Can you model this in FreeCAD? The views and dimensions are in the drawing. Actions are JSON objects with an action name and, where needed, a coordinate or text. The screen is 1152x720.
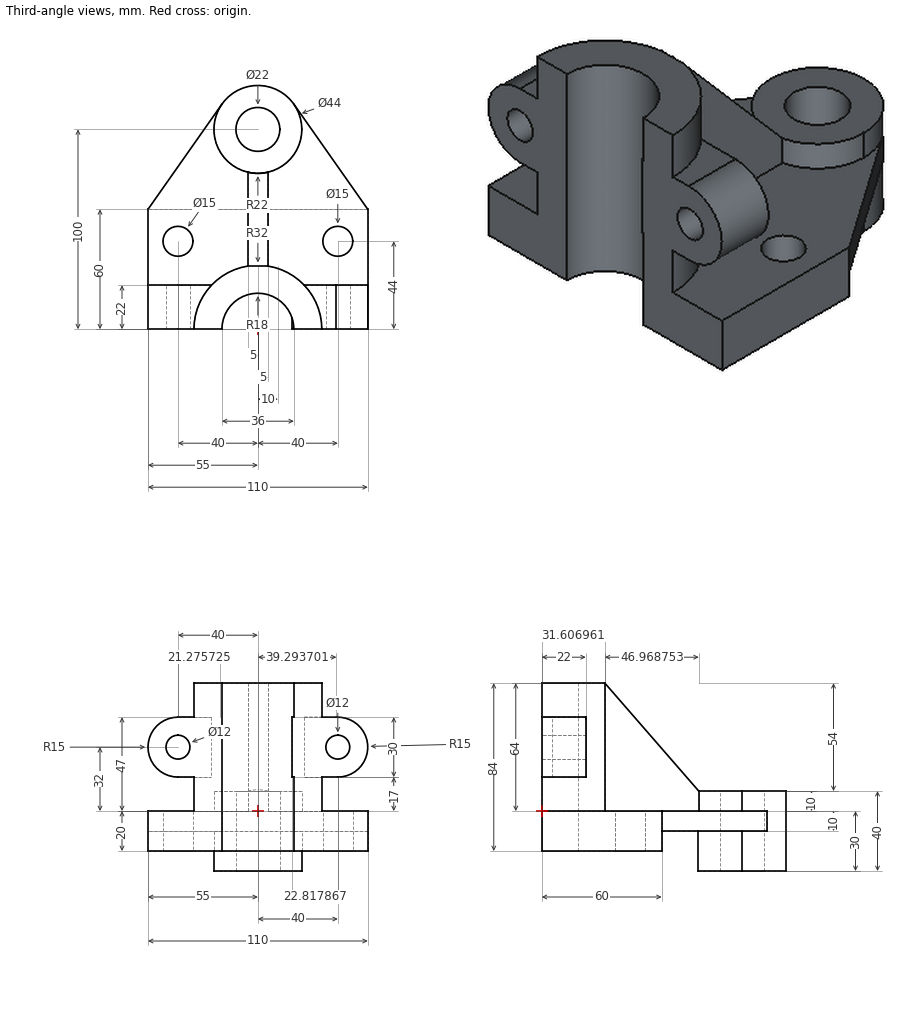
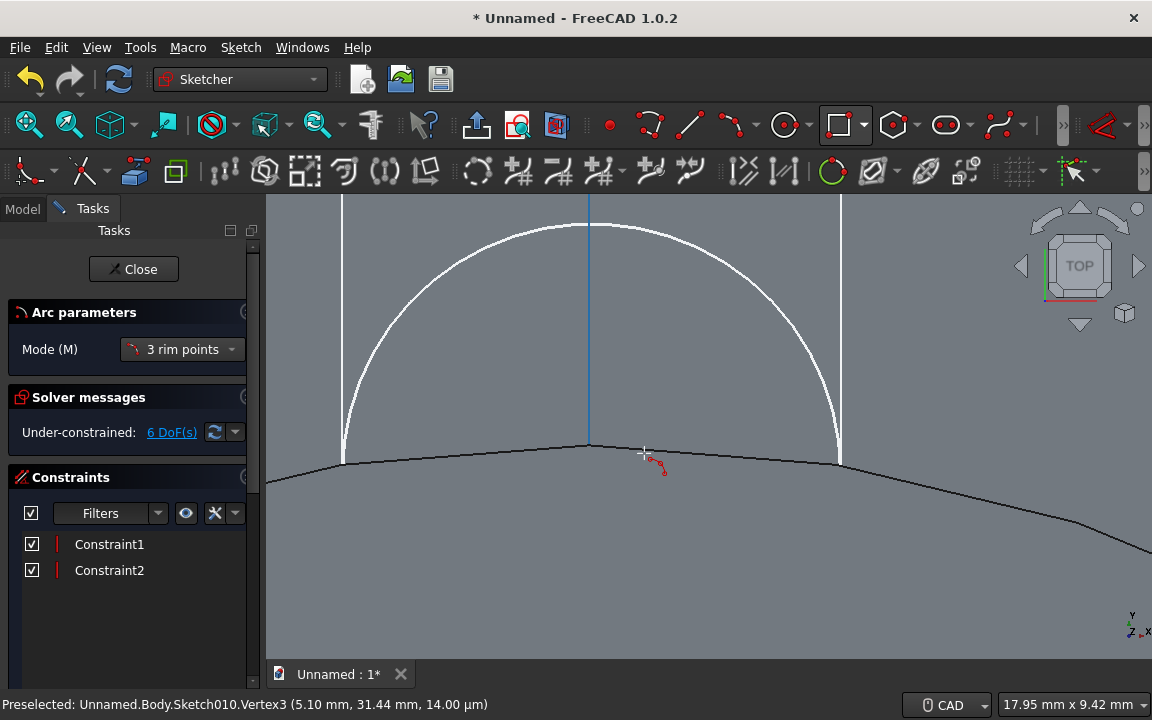
{"action": "left_click", "coordinate": [639, 446]}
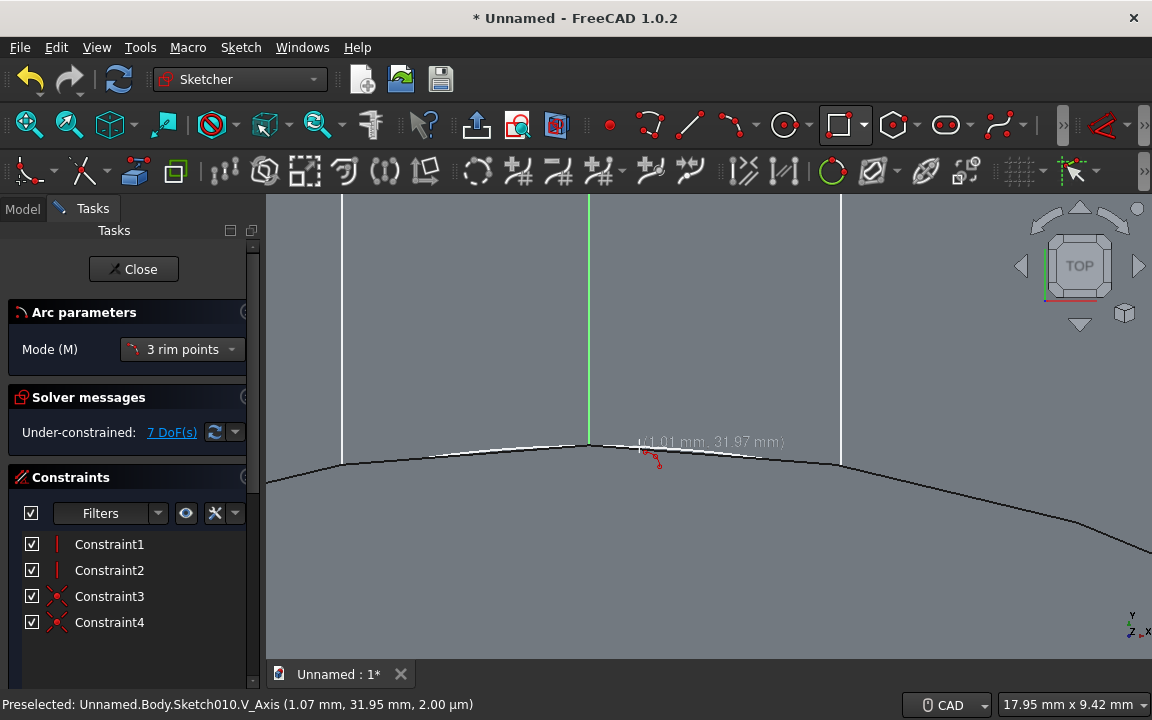
{"action": "scroll", "coordinate": [645, 454], "scroll_direction": "down", "scroll_amount": 13}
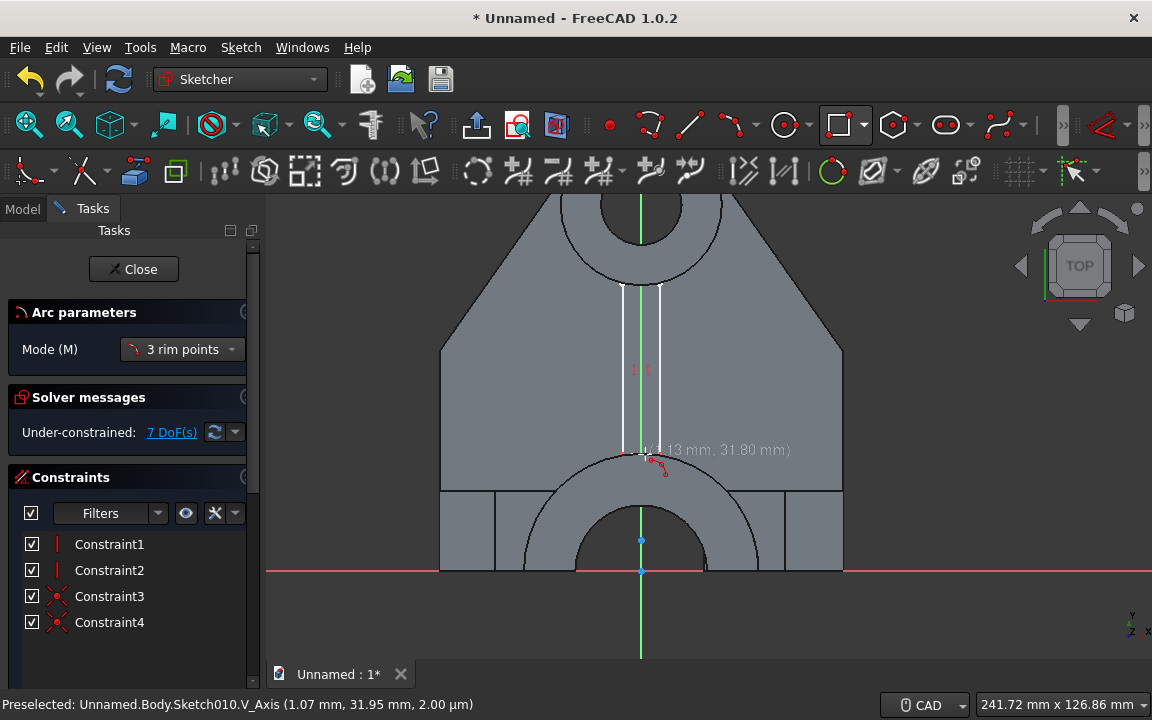
{"action": "left_click", "coordinate": [660, 284]}
{"action": "left_click", "coordinate": [623, 284]}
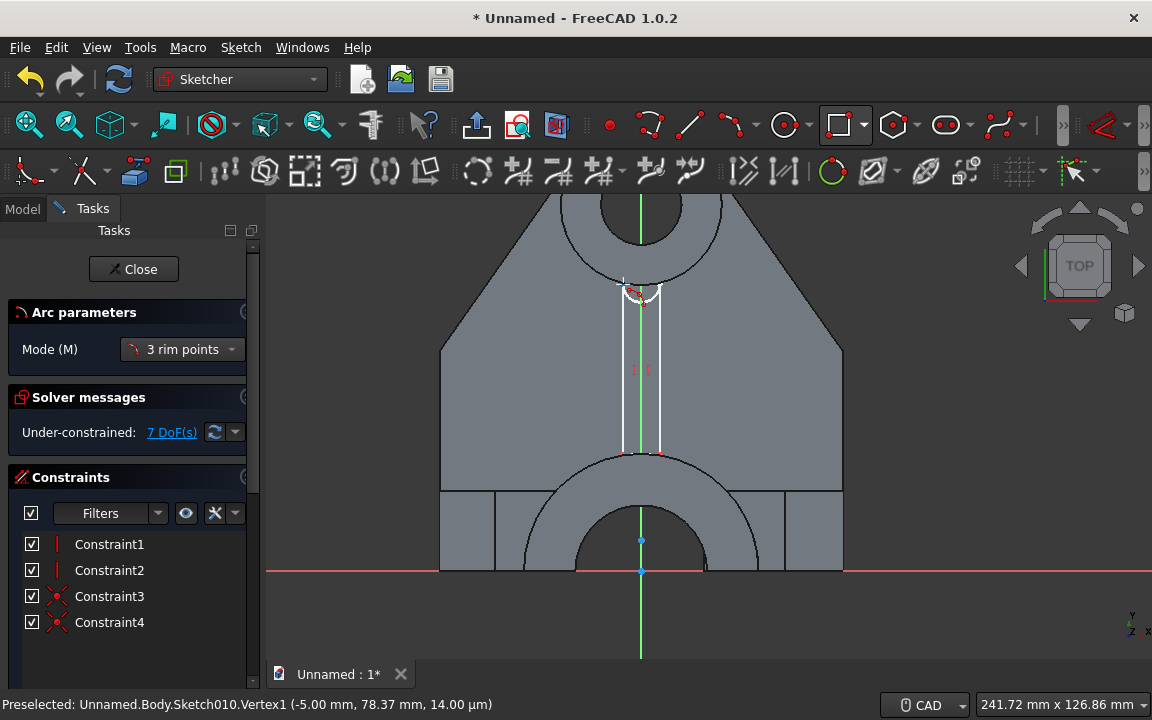
{"action": "scroll", "coordinate": [638, 285], "scroll_direction": "up", "scroll_amount": 11}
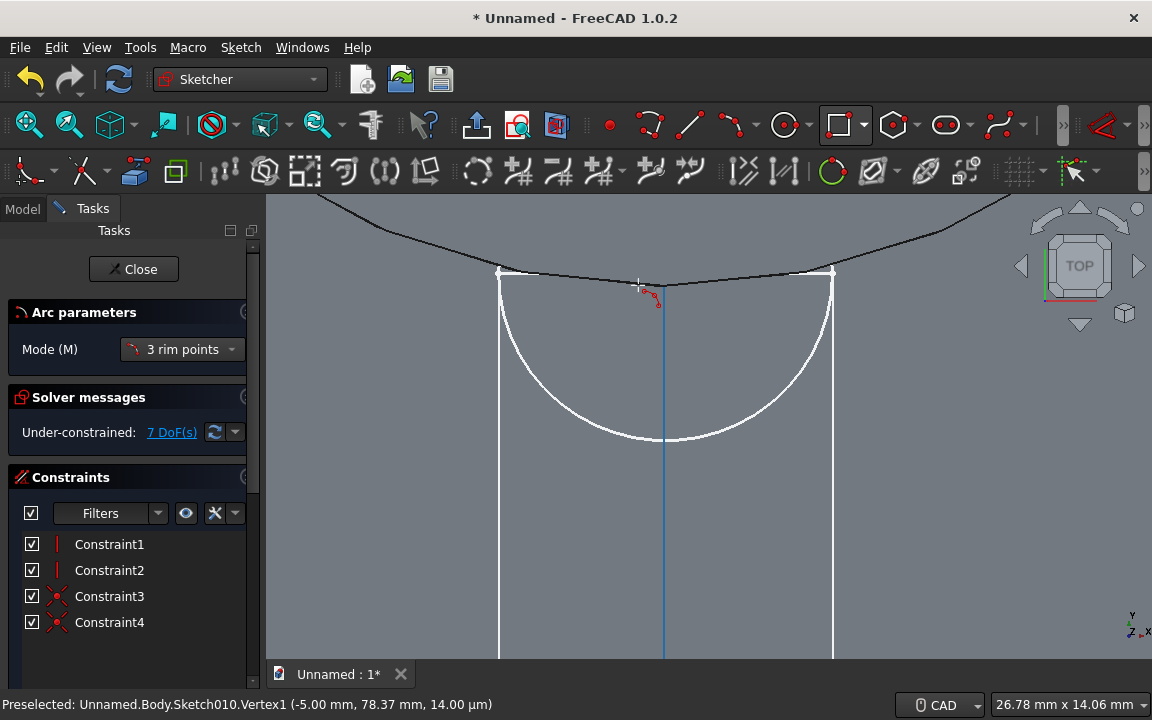
{"action": "left_click", "coordinate": [631, 285]}
{"action": "key", "text": "Escape"}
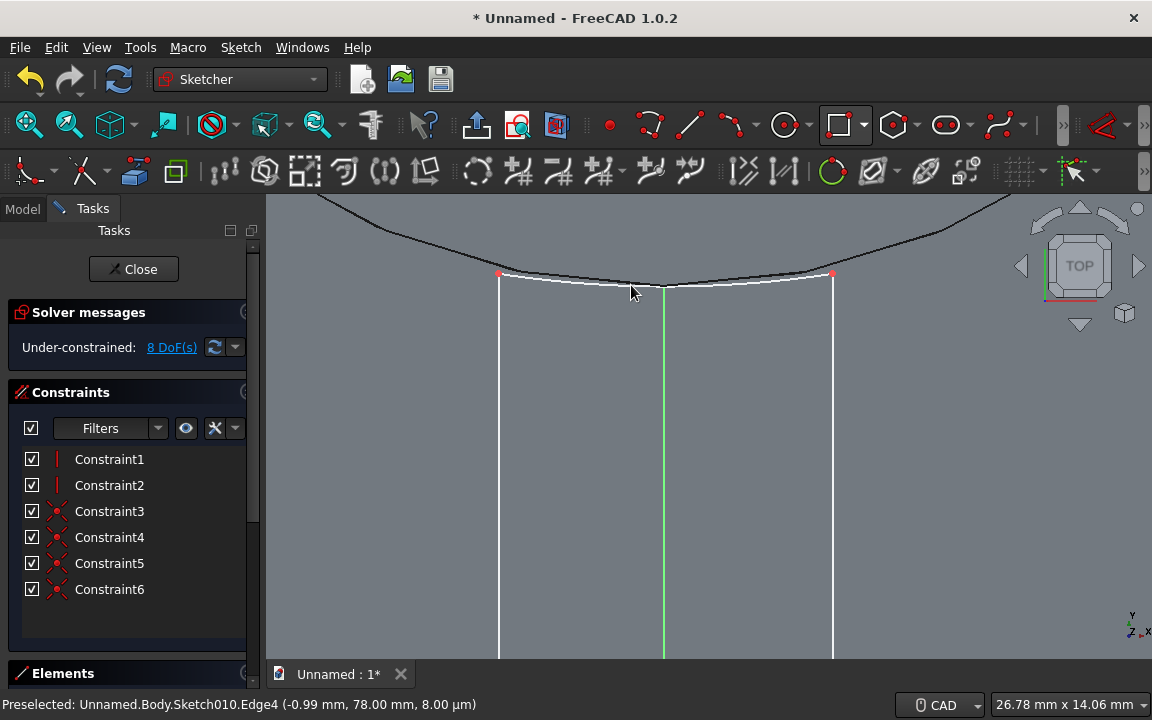
{"action": "scroll", "coordinate": [638, 284], "scroll_direction": "down", "scroll_amount": 11}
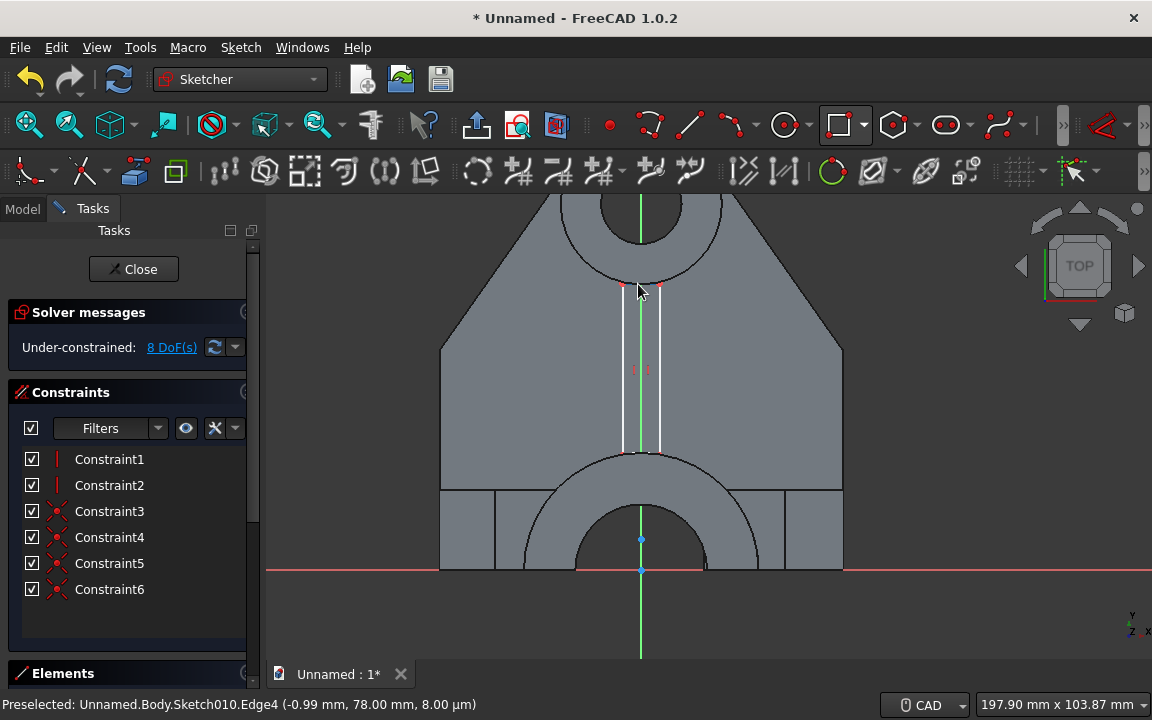
{"action": "left_click_drag", "start_coordinate": [631, 530], "coordinate": [651, 580]}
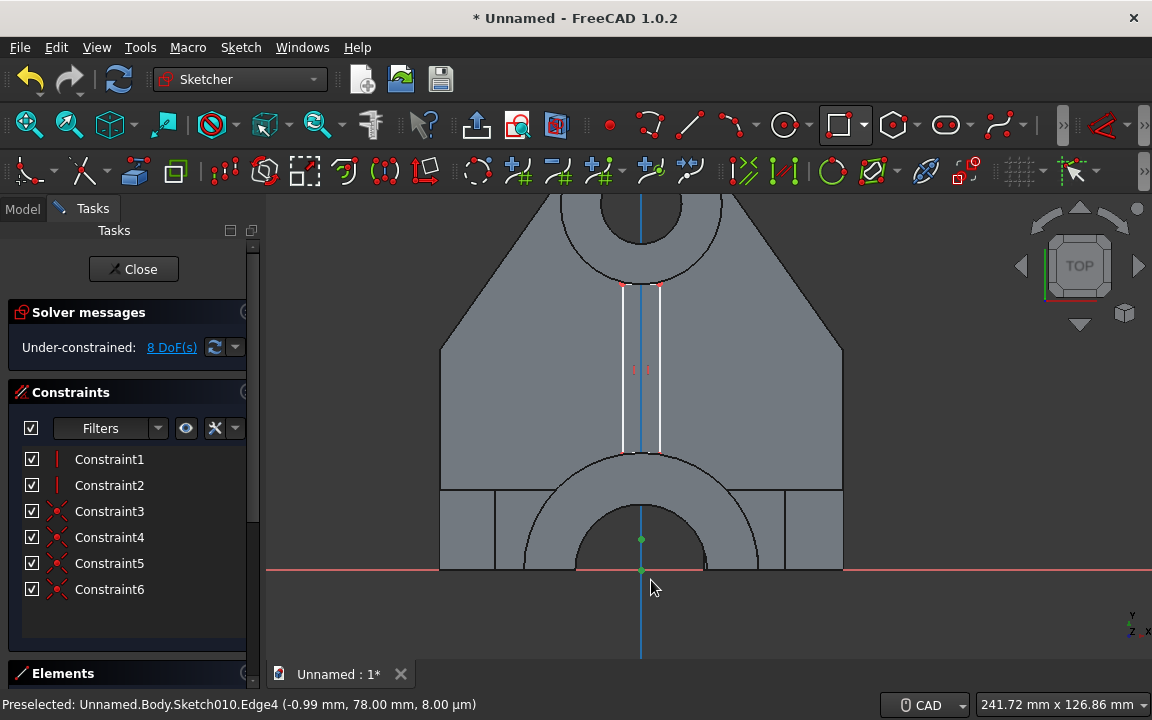
{"action": "key", "text": "c"}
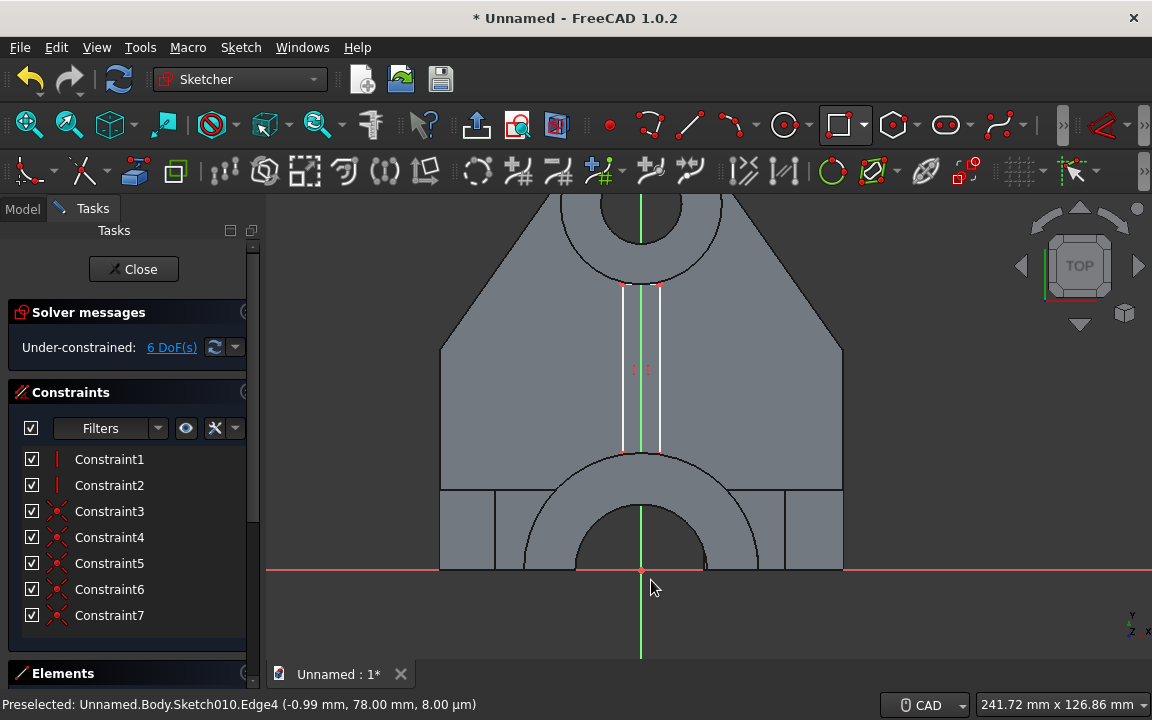
{"action": "scroll", "coordinate": [639, 548], "scroll_direction": "down", "scroll_amount": 2}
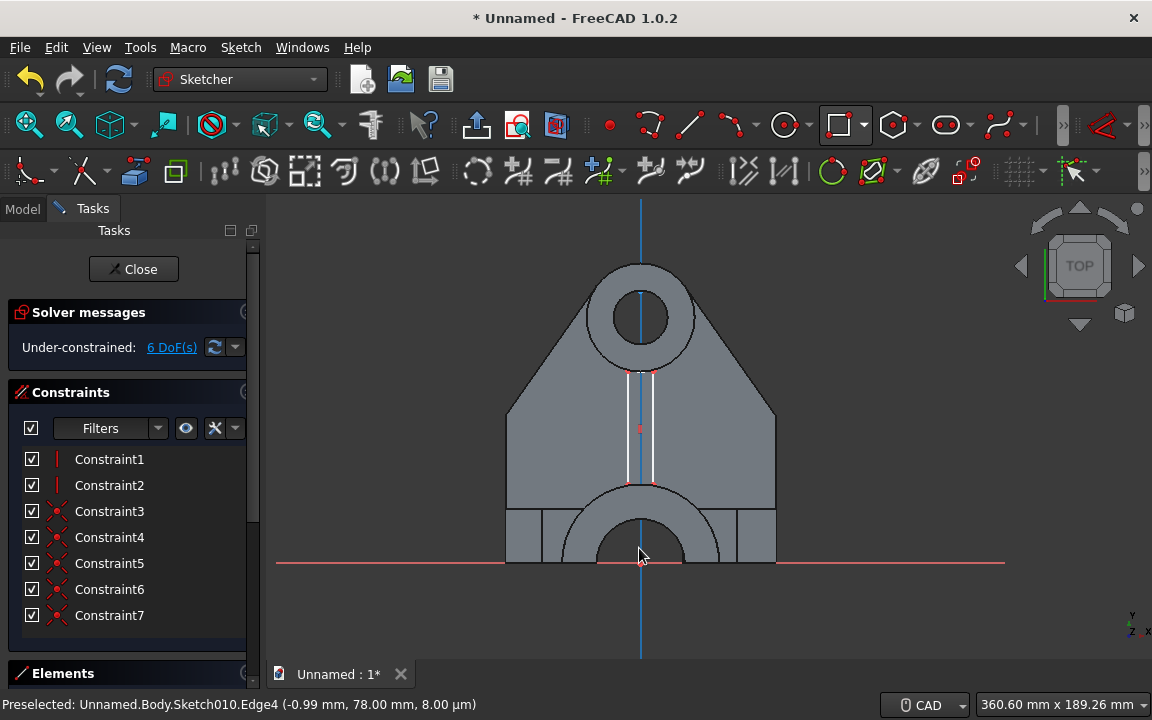
{"action": "left_click", "coordinate": [641, 290]}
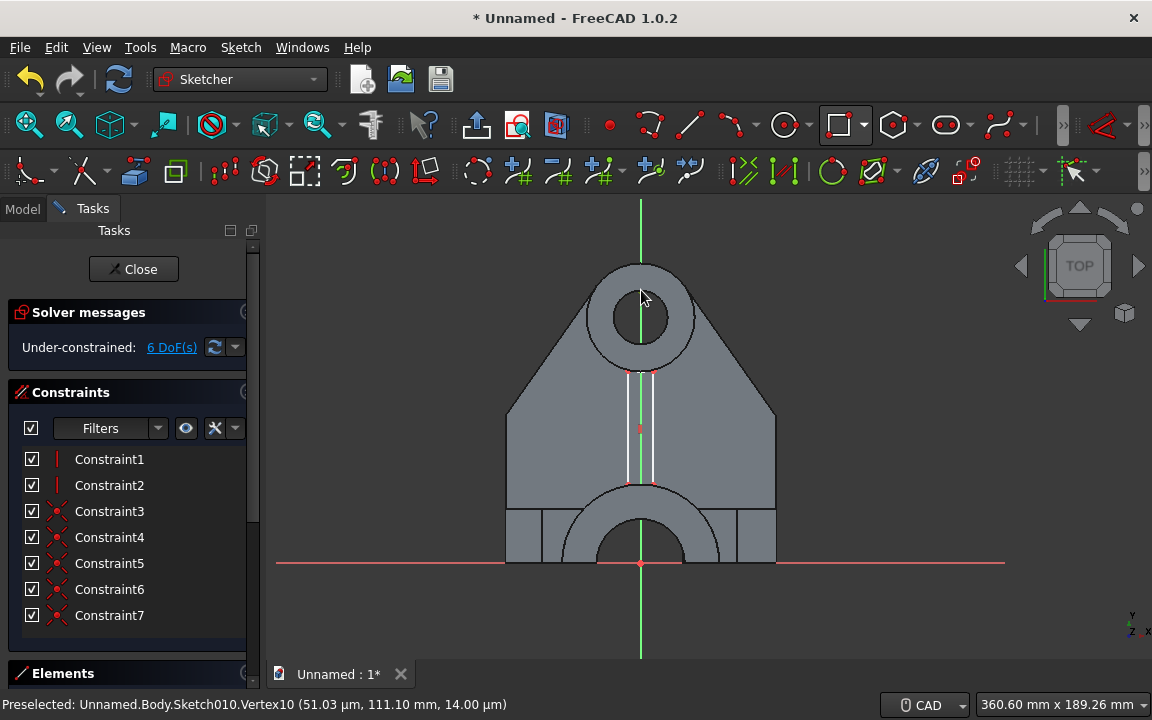
{"action": "left_click", "coordinate": [641, 602]}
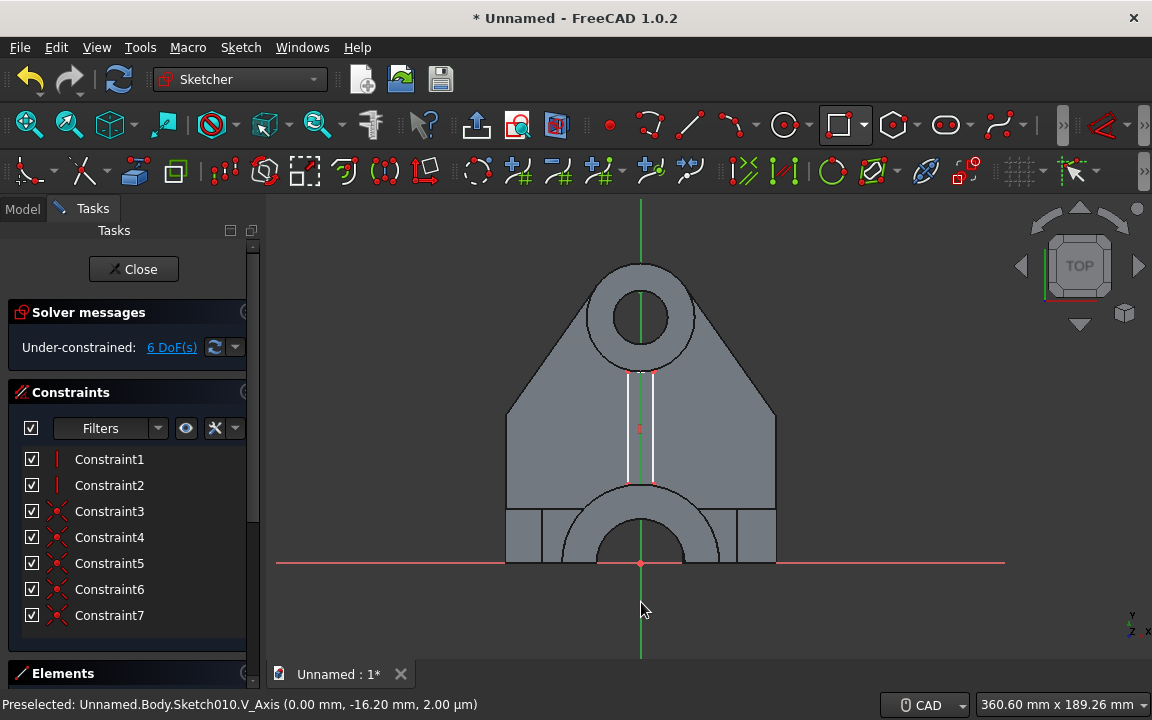
{"action": "key", "text": "c"}